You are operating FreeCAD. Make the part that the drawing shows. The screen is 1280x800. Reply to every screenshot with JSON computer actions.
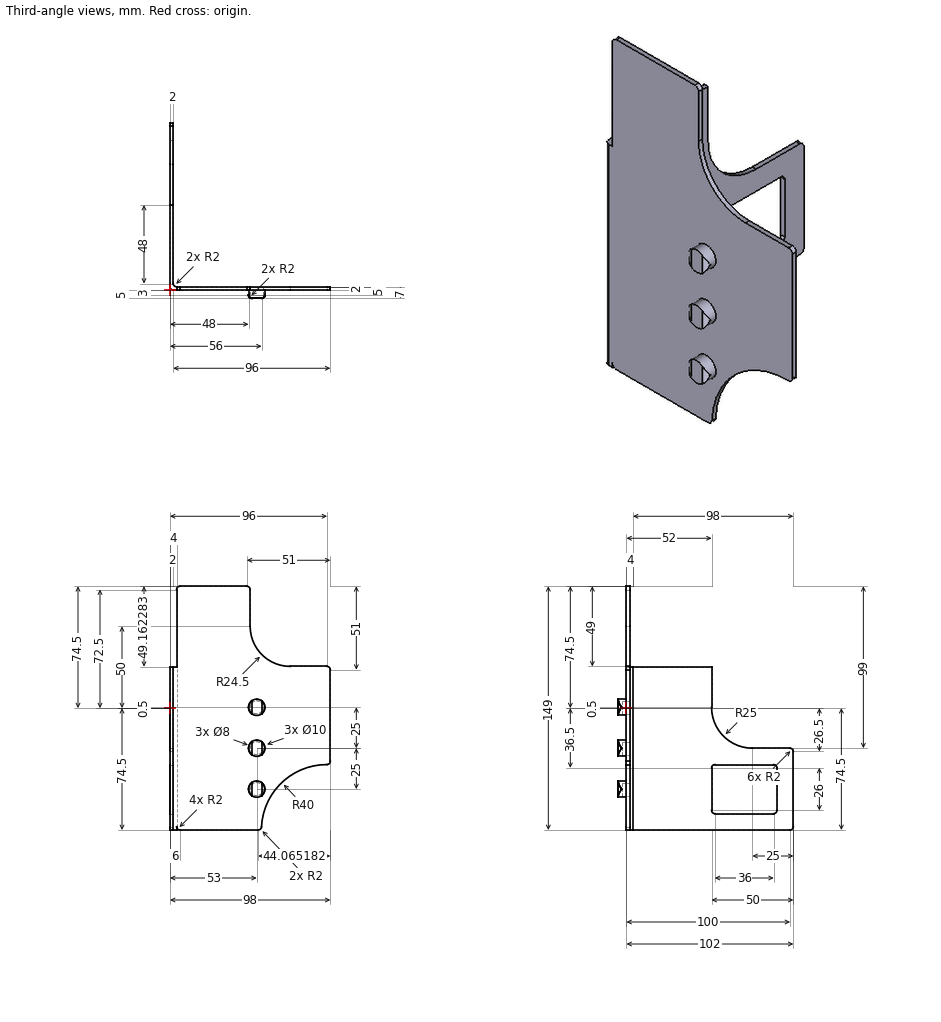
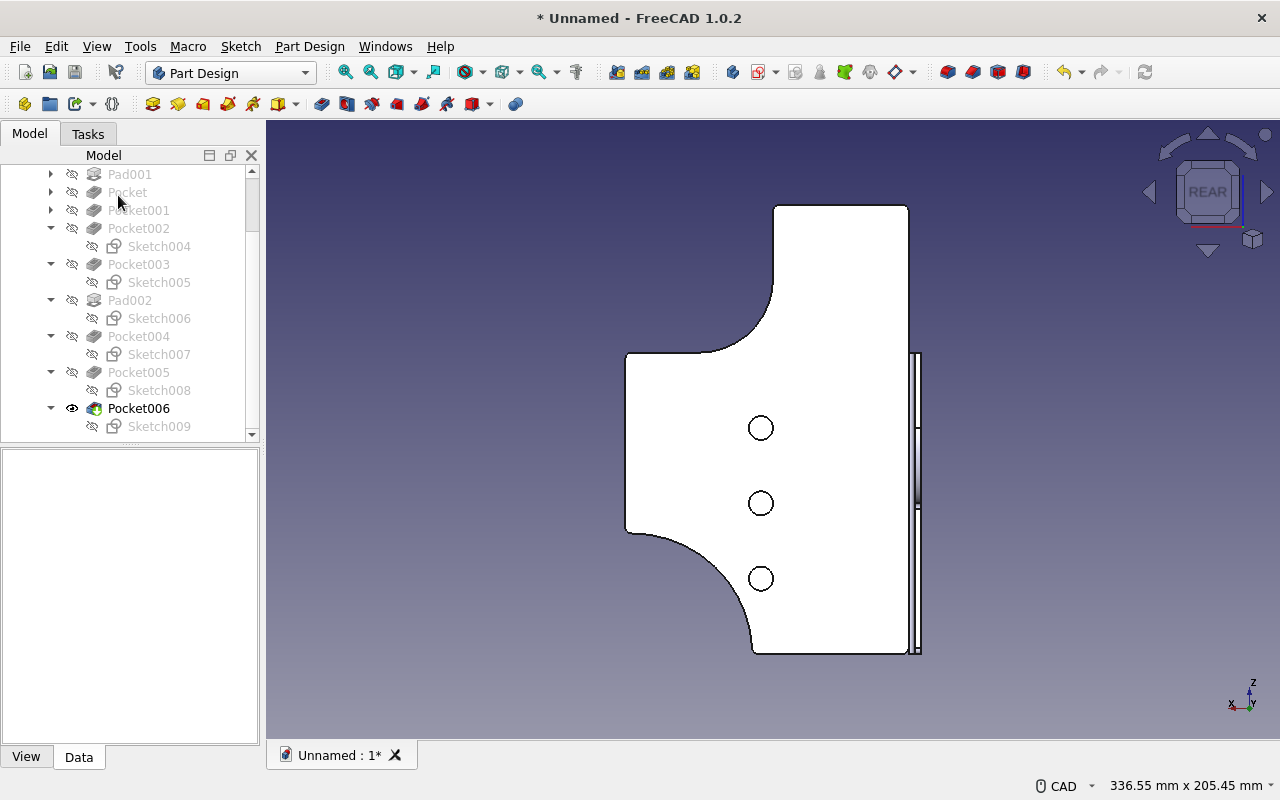
{"action": "key", "text": "0"}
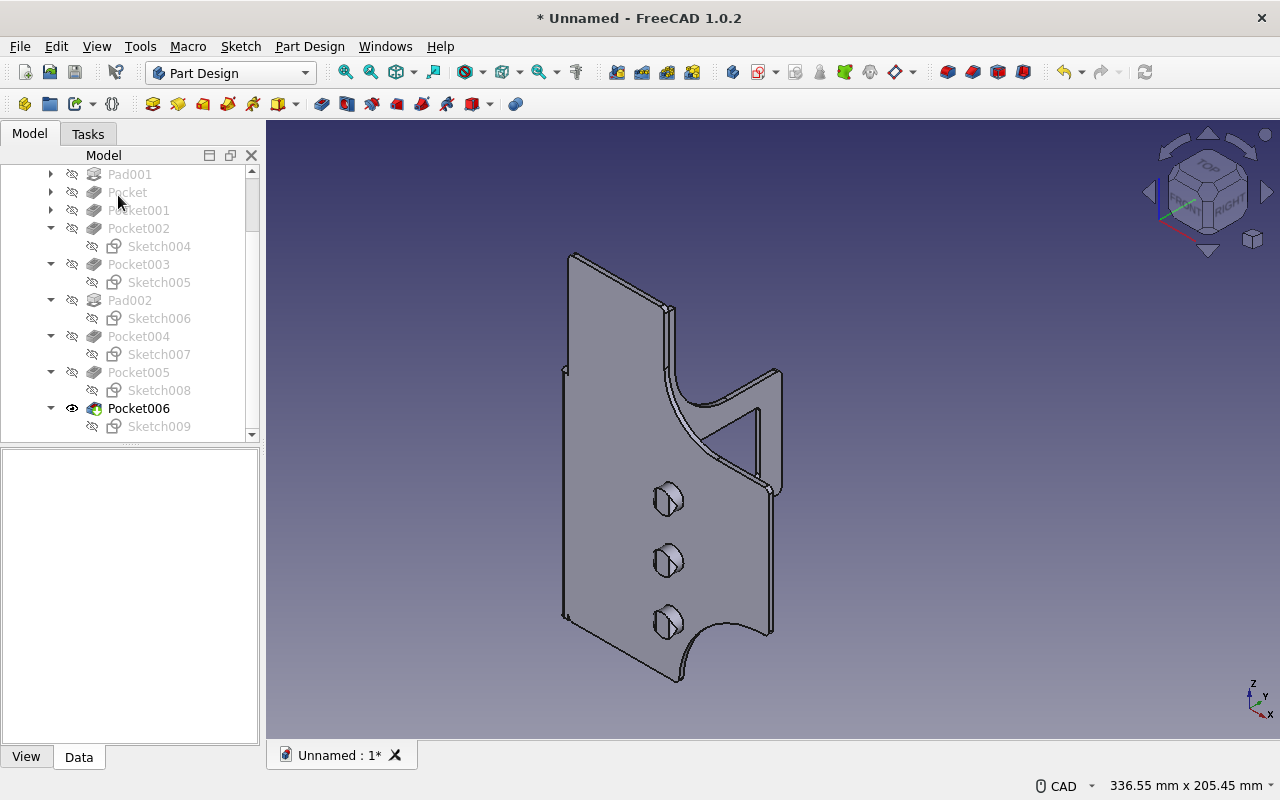
{"action": "key", "text": "v f"}